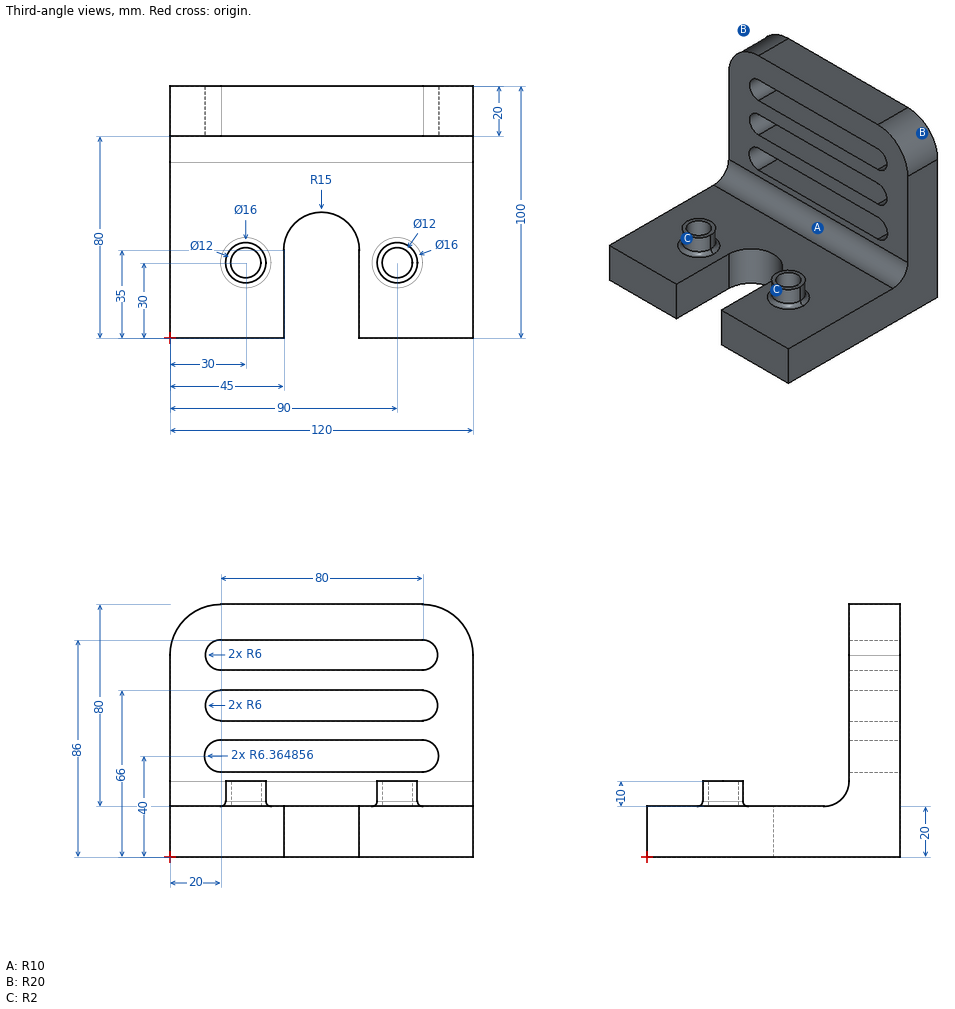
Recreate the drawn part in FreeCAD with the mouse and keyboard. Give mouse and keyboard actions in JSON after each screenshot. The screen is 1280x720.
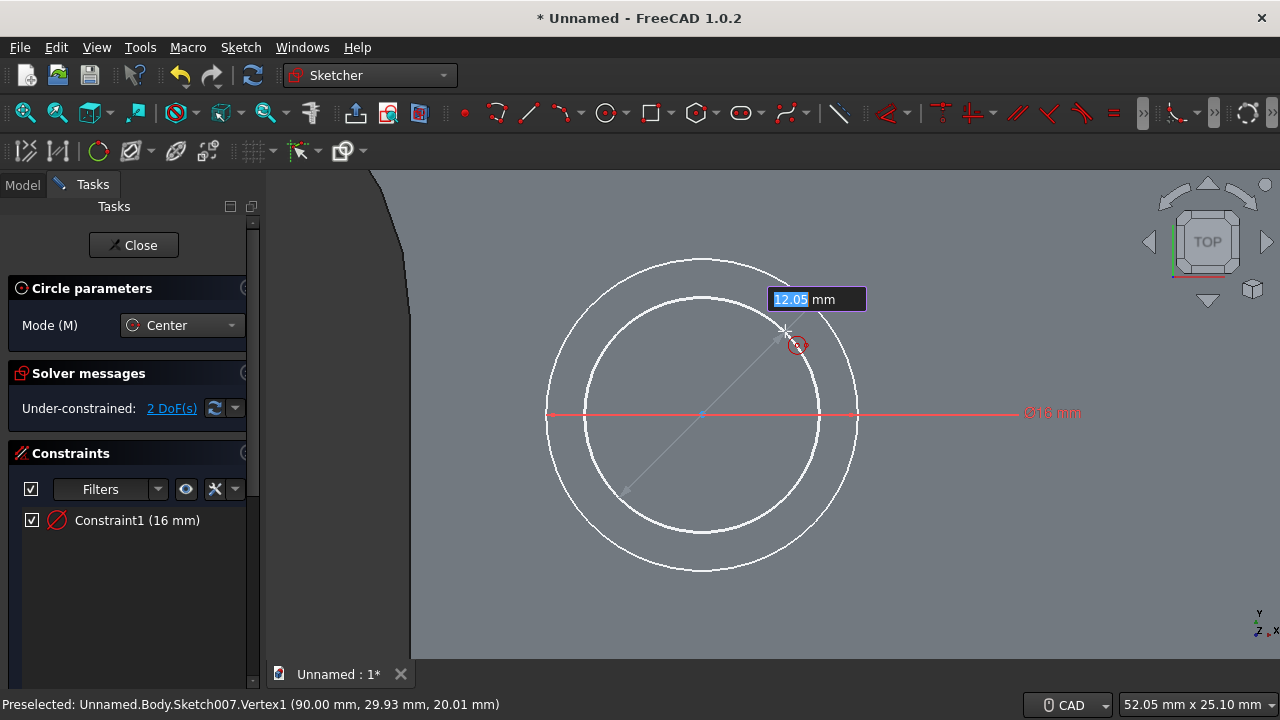
{"action": "type", "text": "12"}
{"action": "key", "text": "Return"}
{"action": "key", "text": "Escape"}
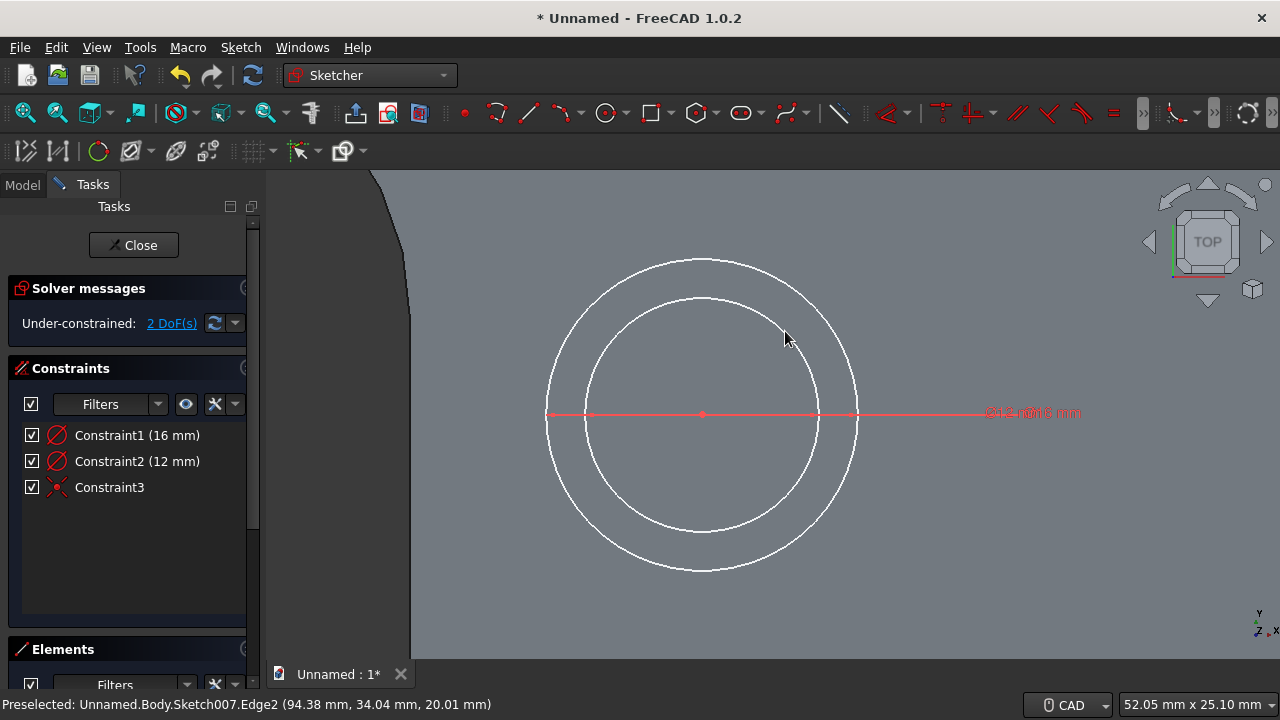
{"action": "left_click", "coordinate": [886, 114]}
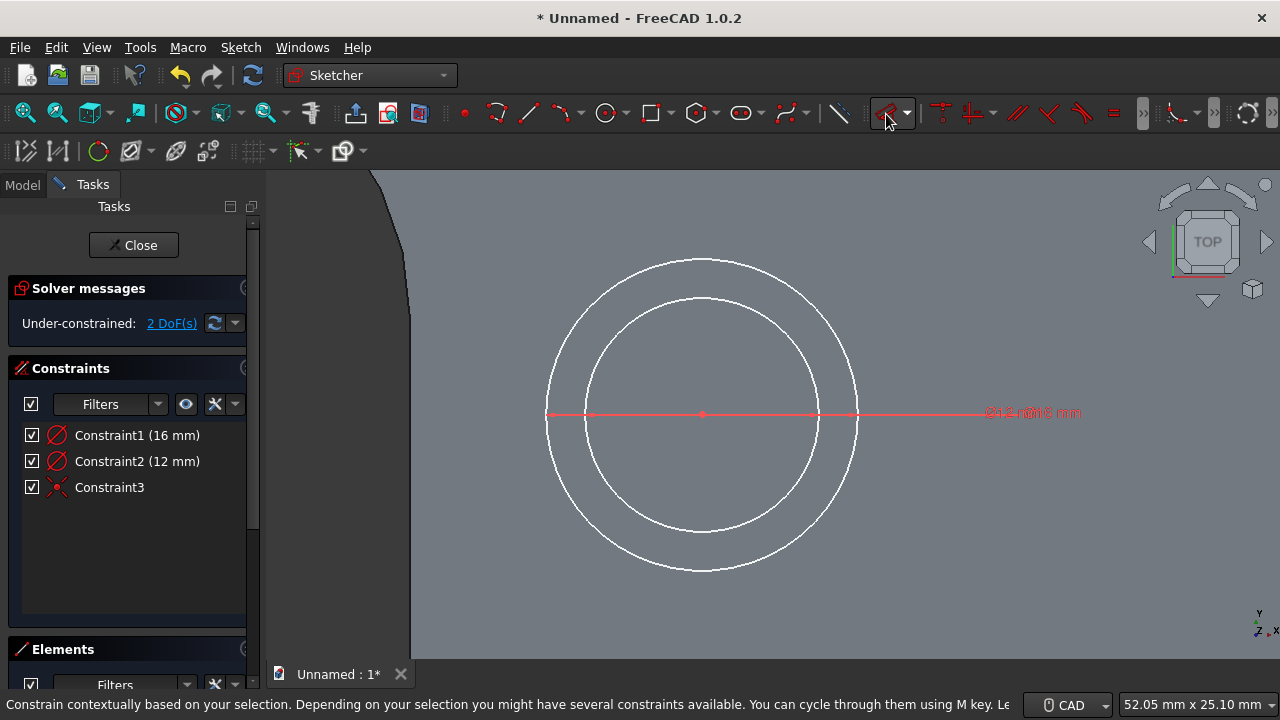
{"action": "left_click", "coordinate": [702, 415]}
{"action": "left_click", "coordinate": [498, 381]}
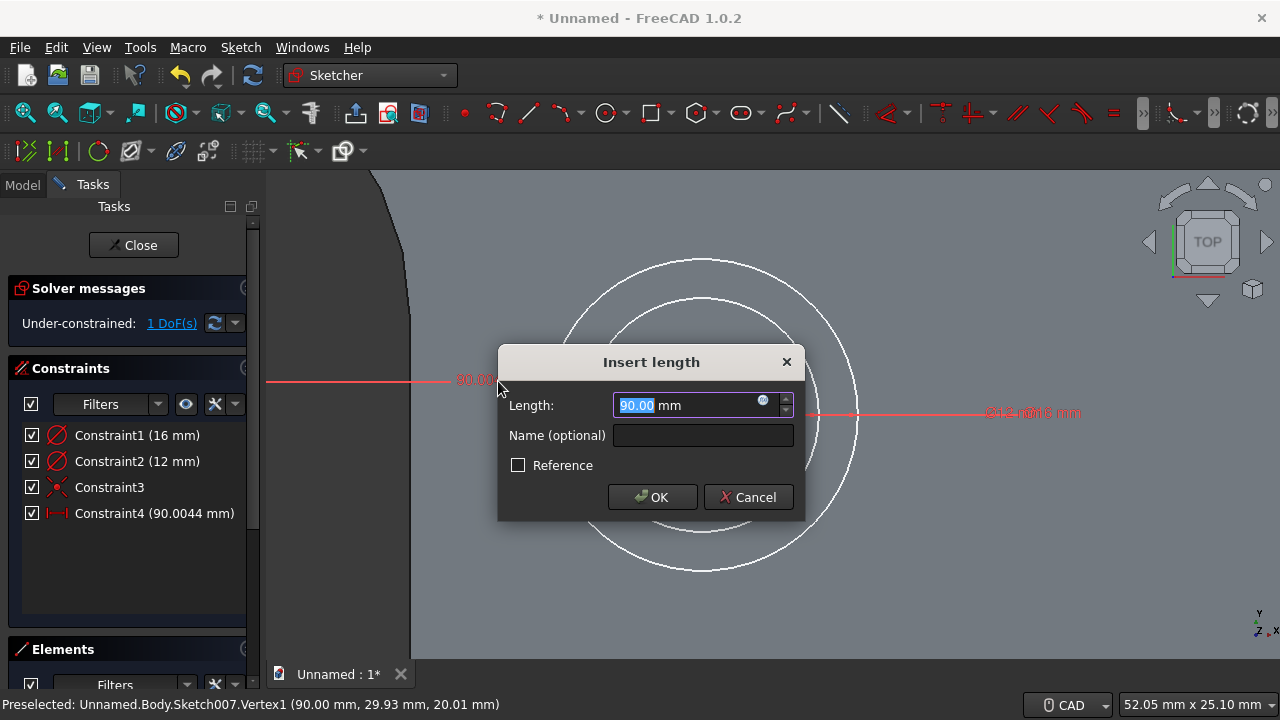
{"action": "type", "text": "90"}
{"action": "key", "text": "Return"}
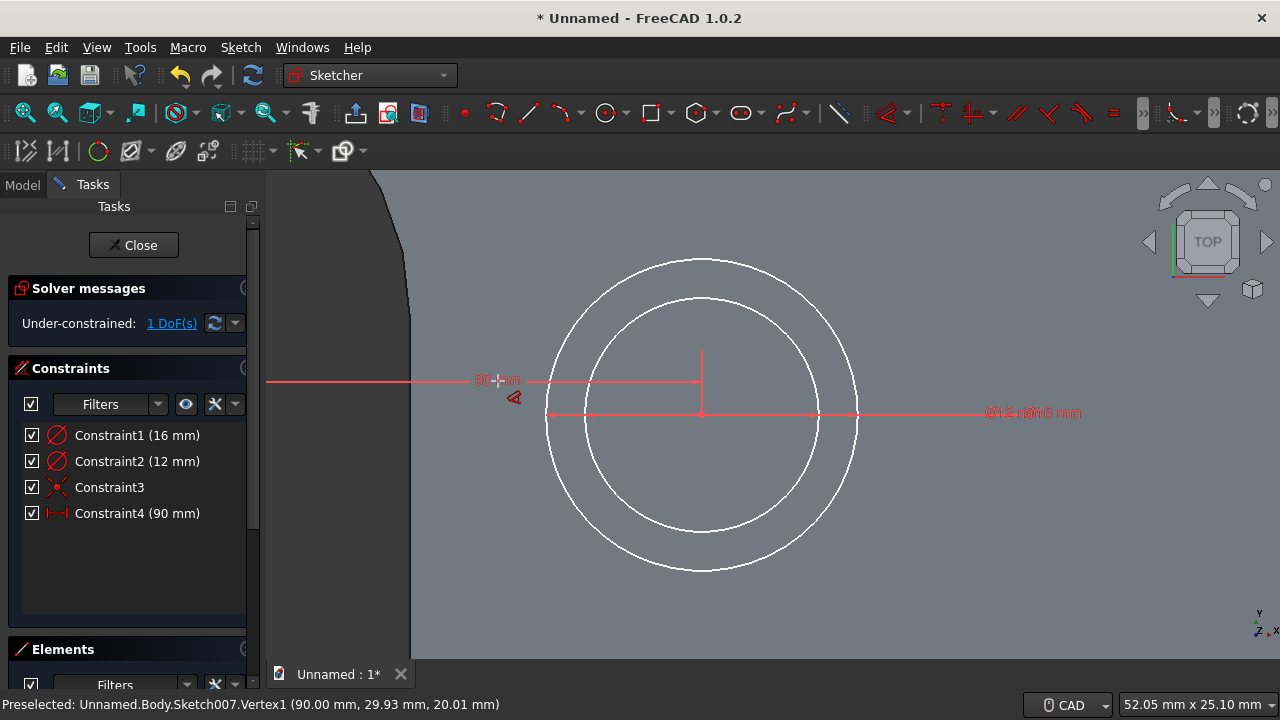
{"action": "left_click", "coordinate": [702, 415]}
{"action": "left_click", "coordinate": [736, 473]}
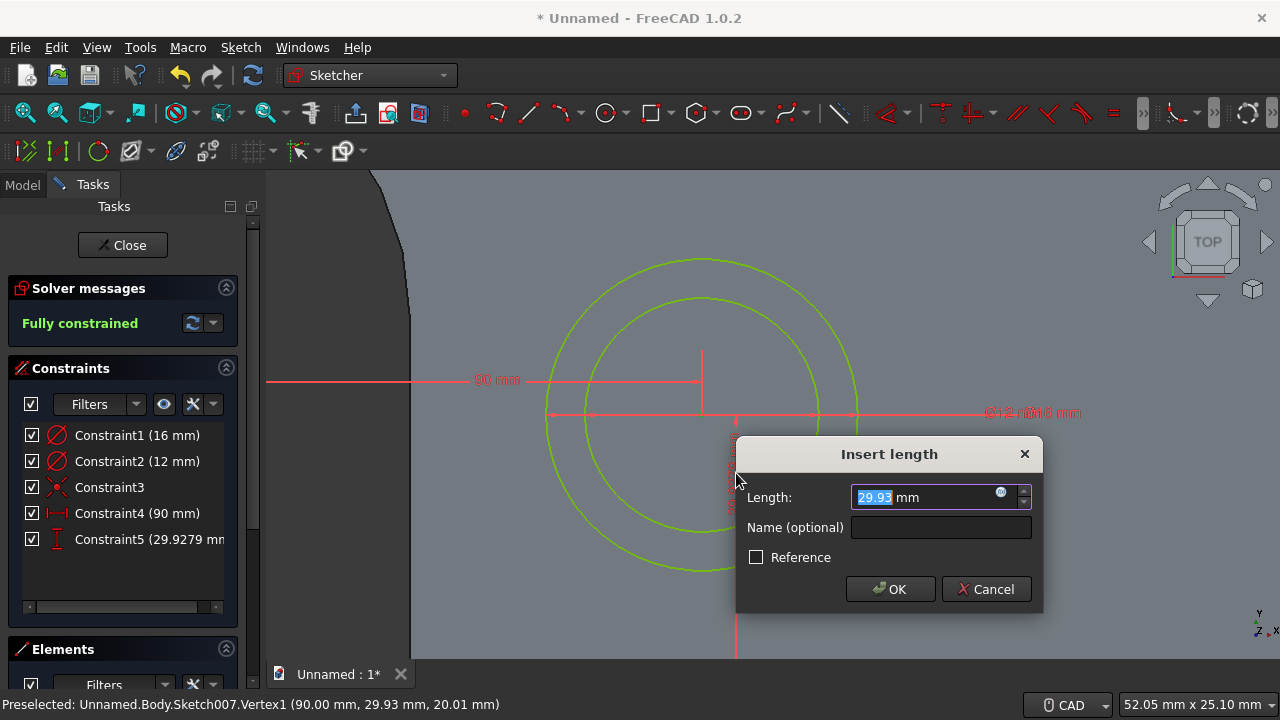
{"action": "type", "text": "30"}
{"action": "key", "text": "Return"}
{"action": "key", "text": "Escape"}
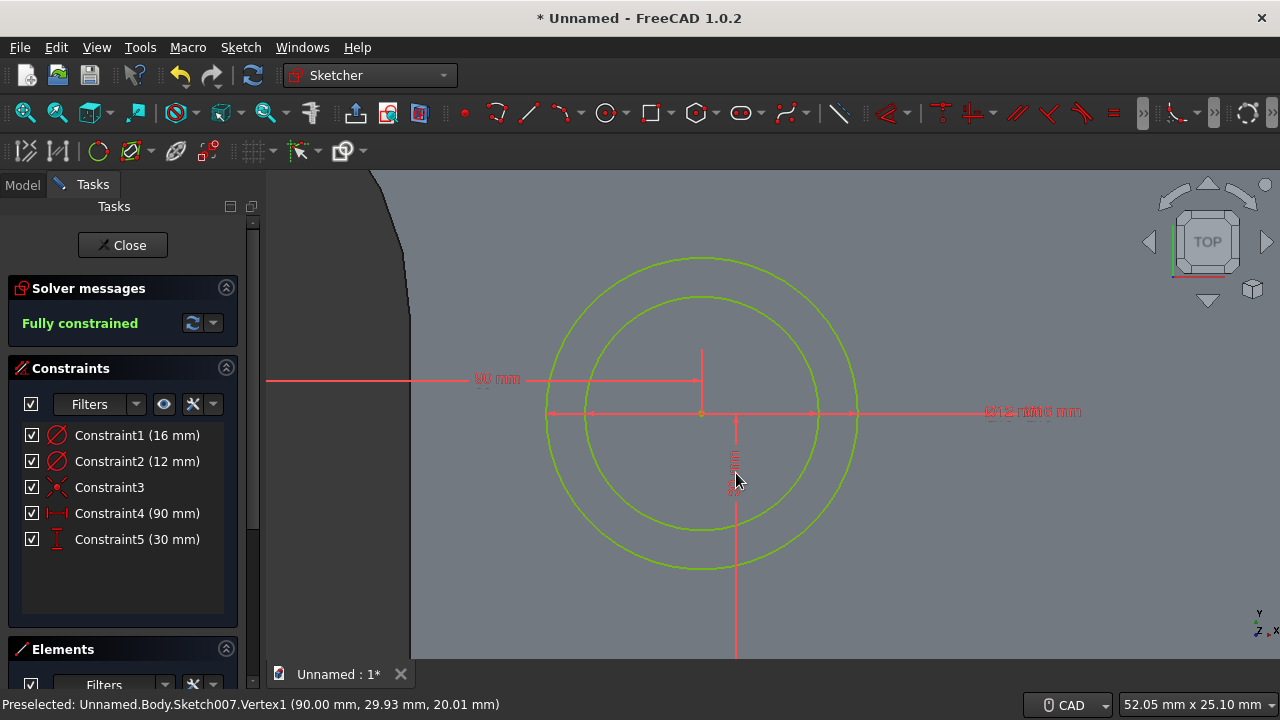
{"action": "left_click", "coordinate": [123, 245]}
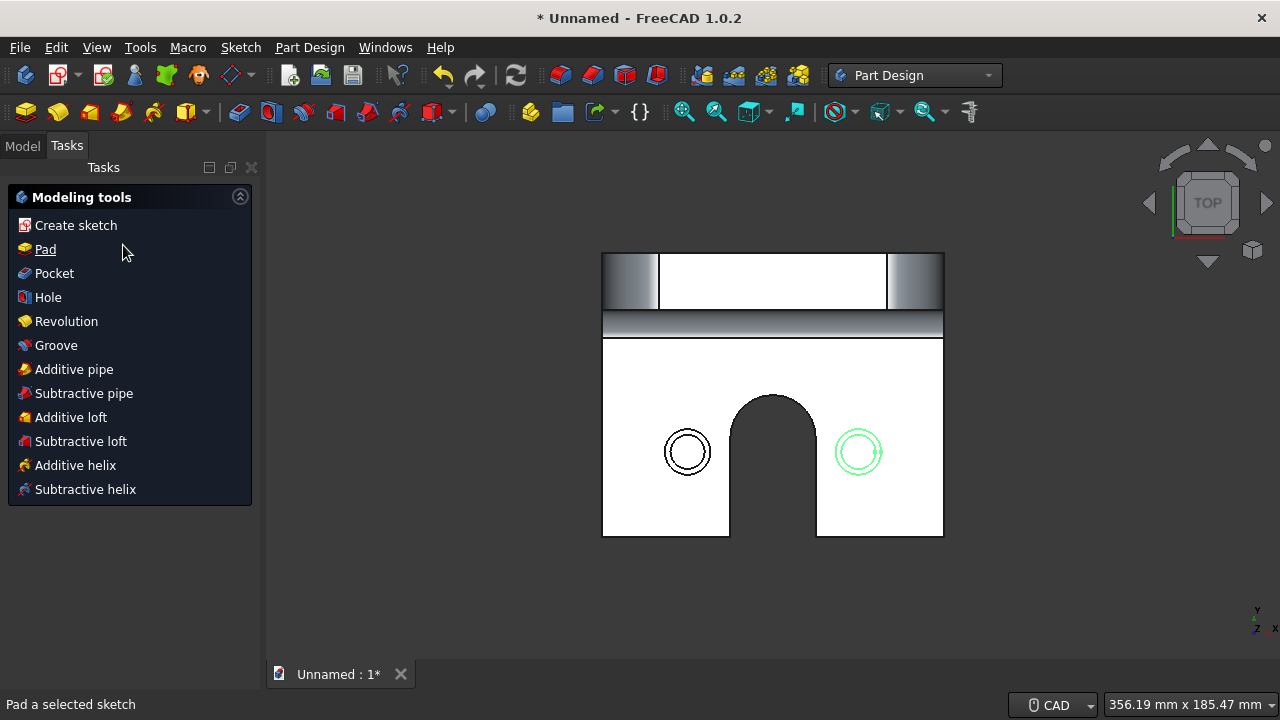
{"action": "left_click", "coordinate": [26, 112]}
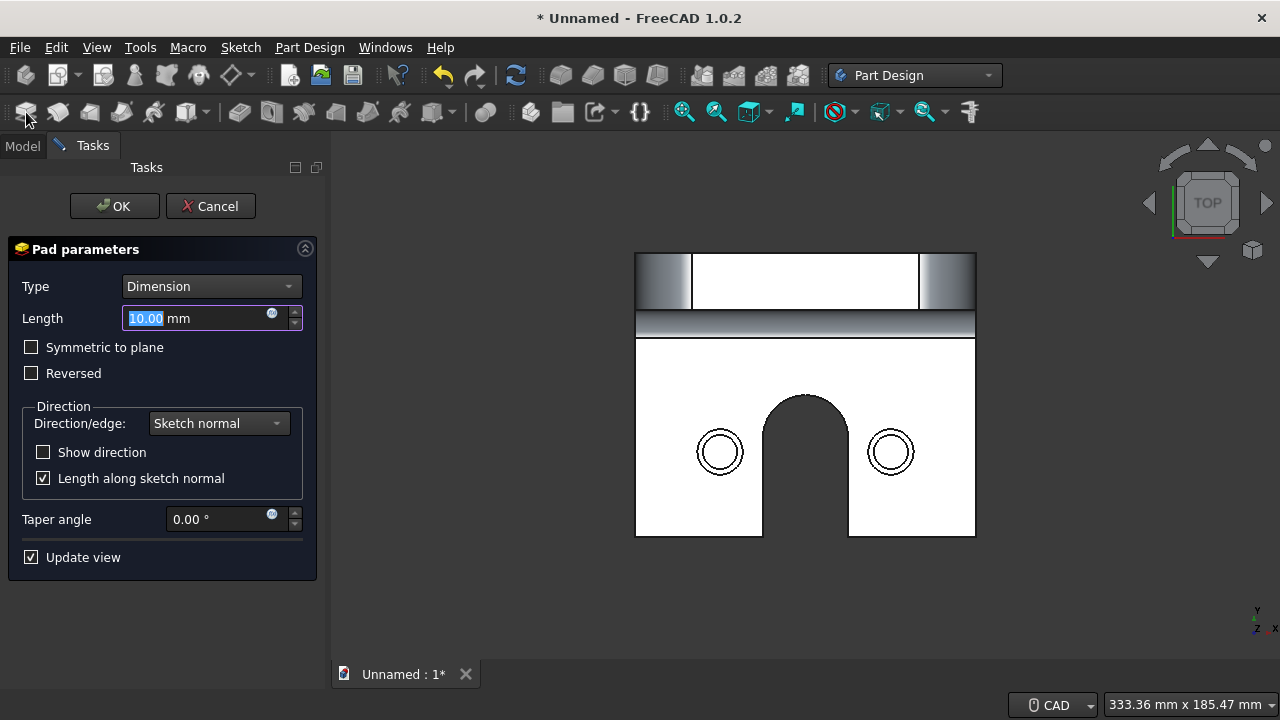
{"action": "type", "text": "10"}
{"action": "key", "text": "Tab"}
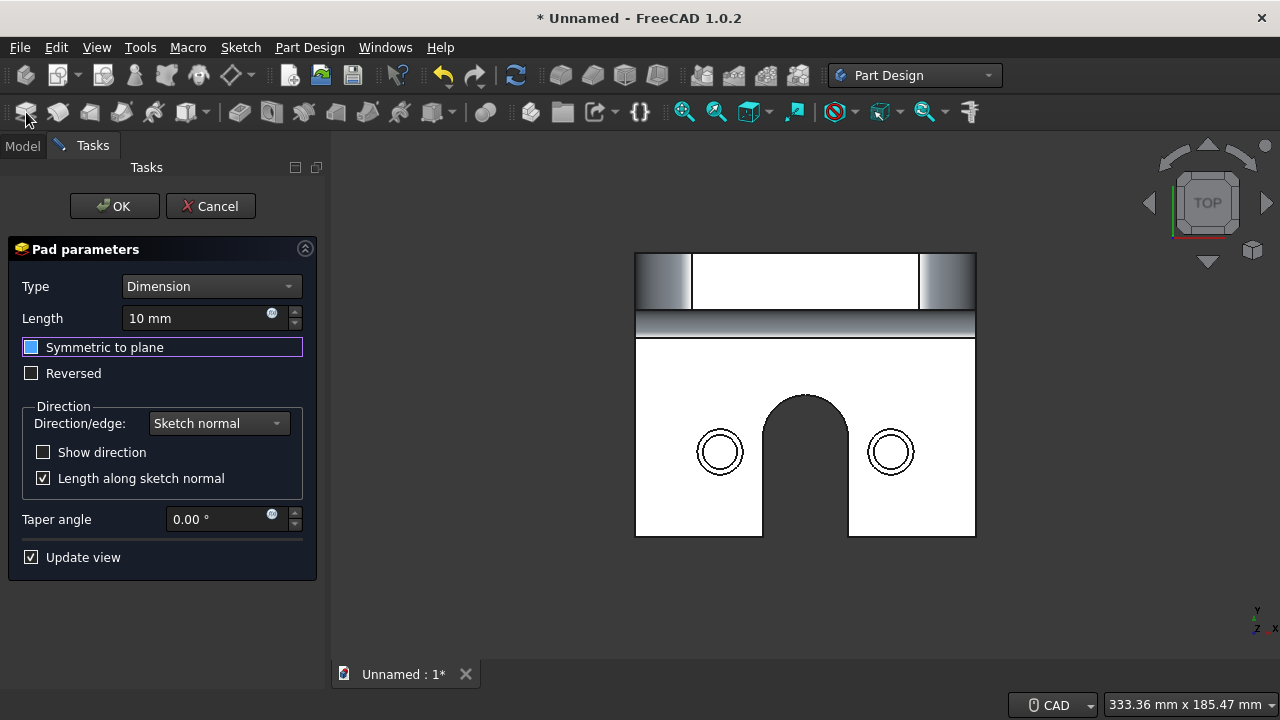
{"action": "left_click", "coordinate": [115, 206]}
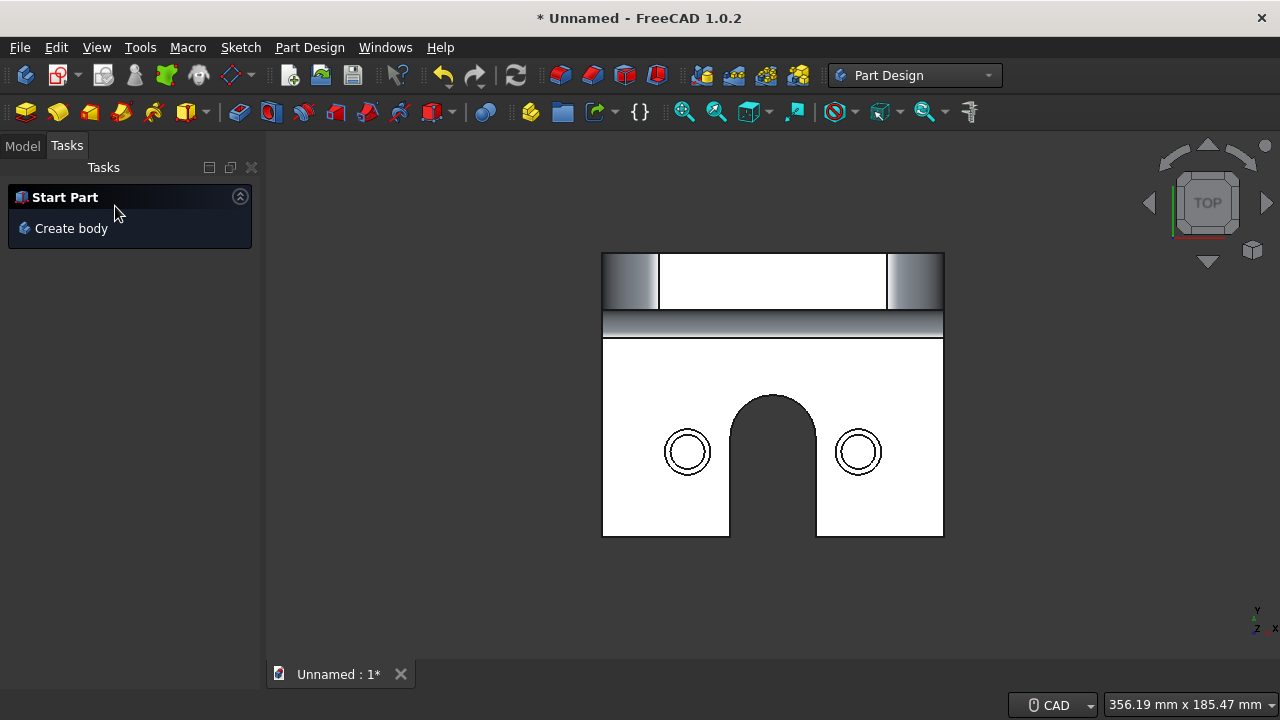
{"action": "key", "text": "0"}